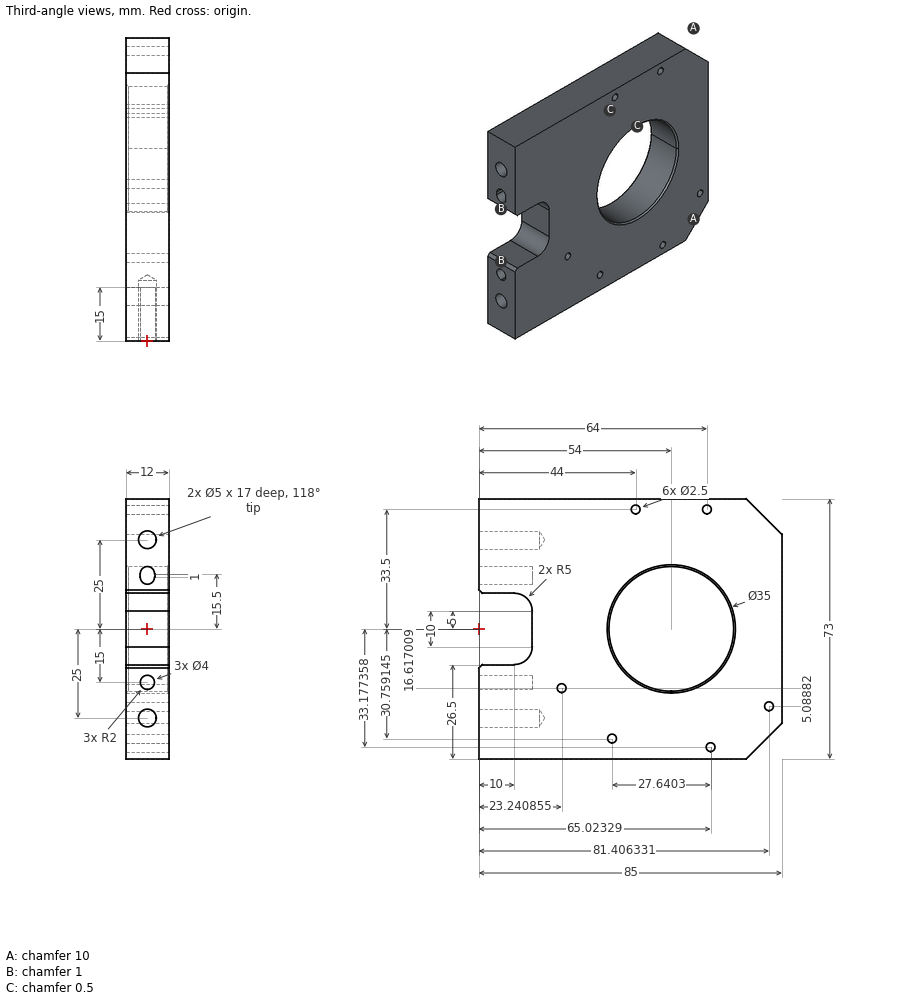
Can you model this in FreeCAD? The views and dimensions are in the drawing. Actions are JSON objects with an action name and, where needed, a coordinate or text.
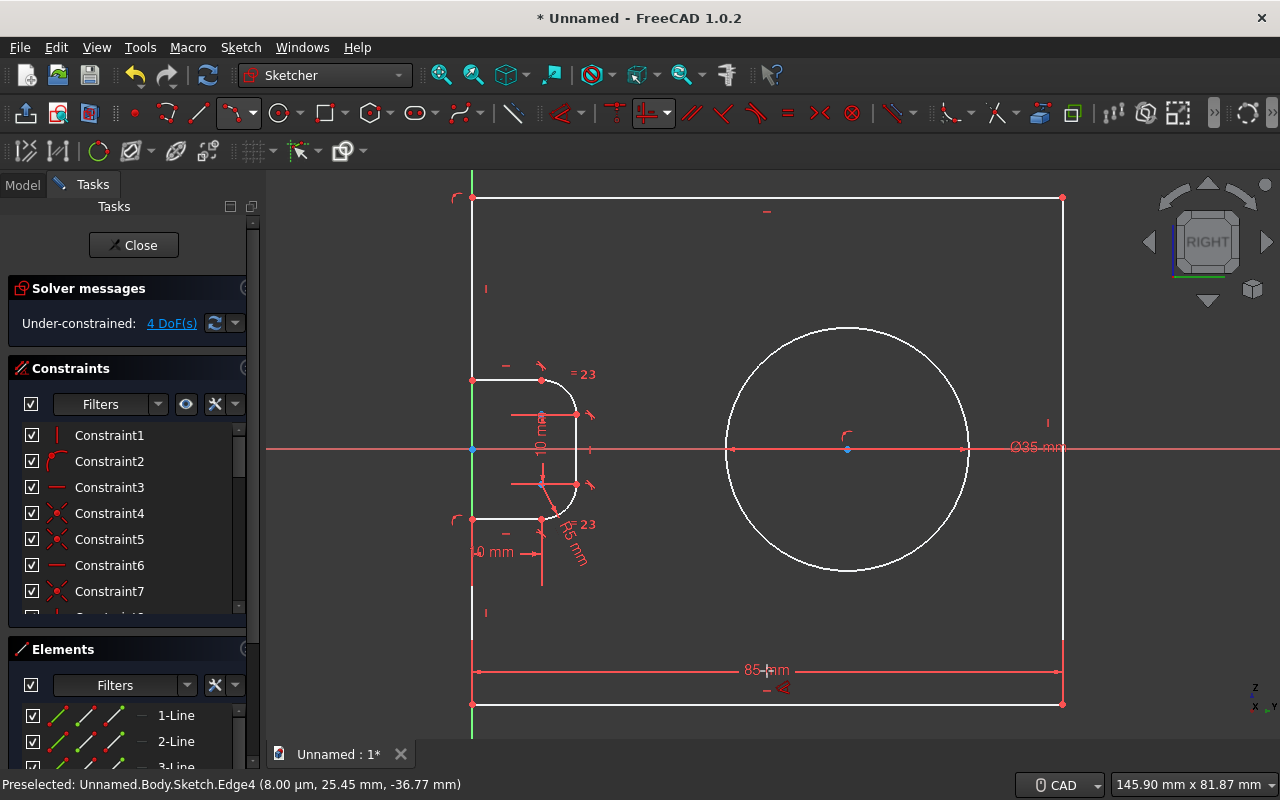
{"action": "left_click", "coordinate": [1063, 553]}
{"action": "left_click", "coordinate": [1097, 335]}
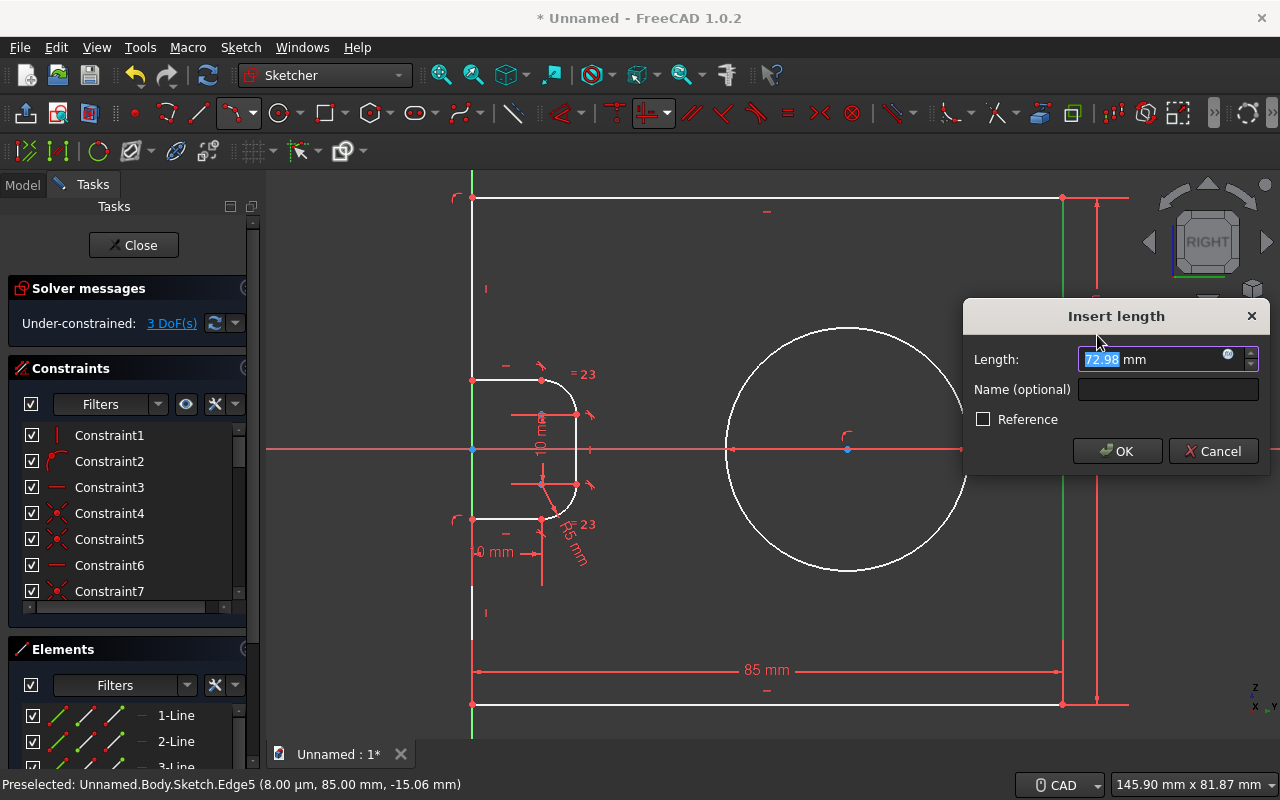
{"action": "type", "text": "73"}
{"action": "key", "text": "Return"}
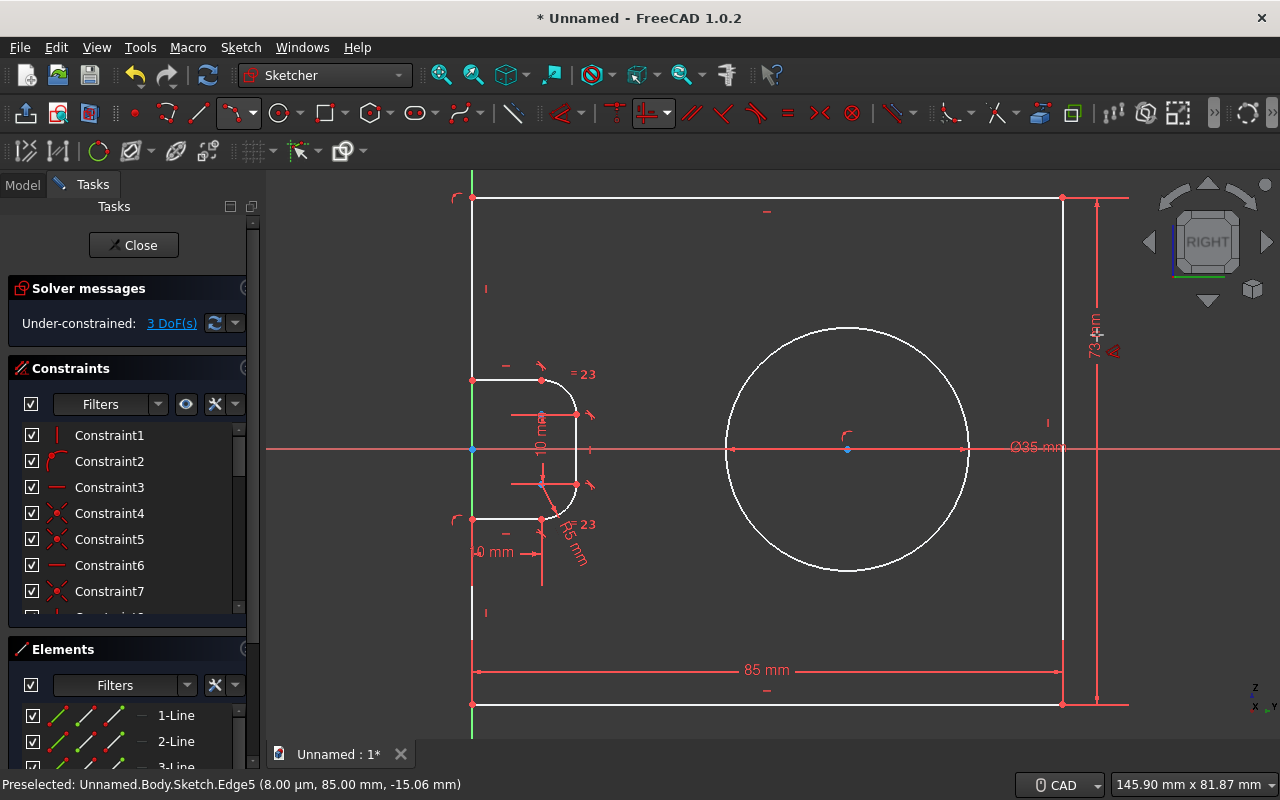
{"action": "left_click", "coordinate": [576, 415]}
{"action": "left_click", "coordinate": [438, 432]}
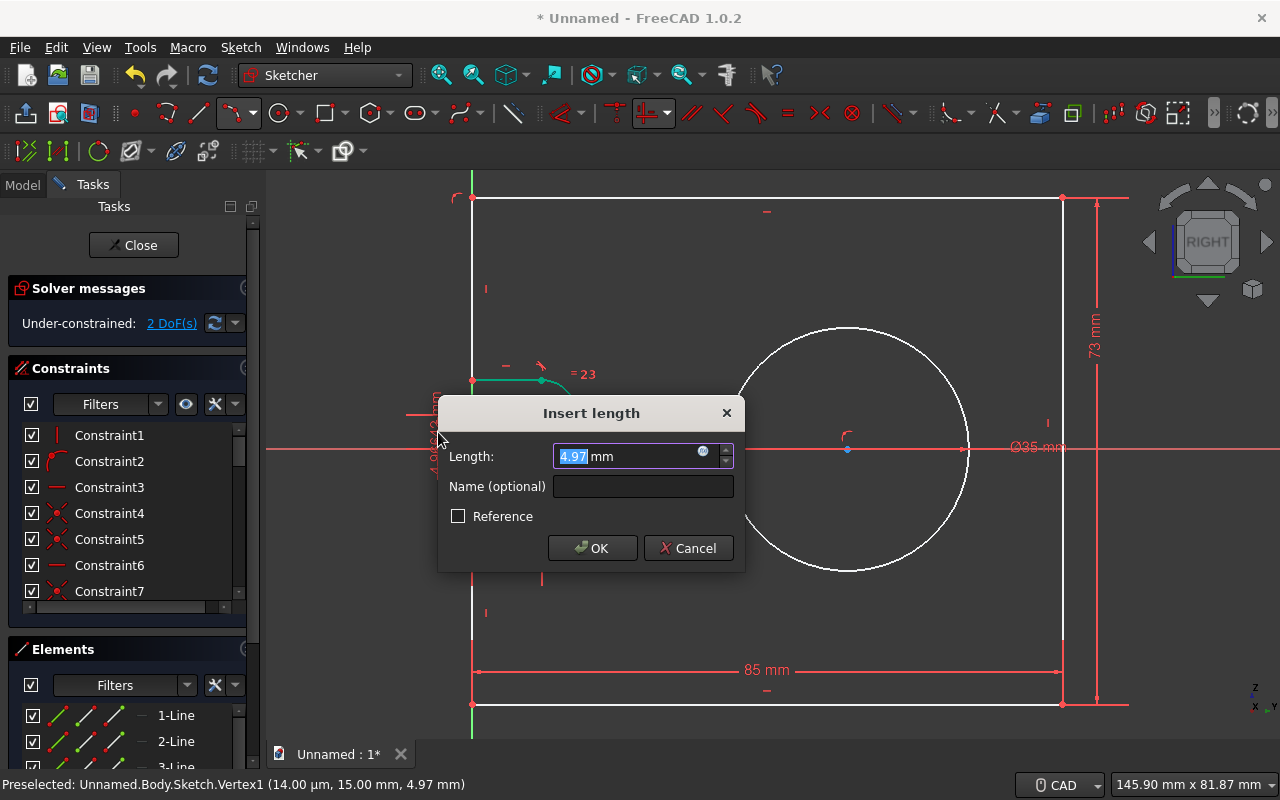
{"action": "type", "text": "5"}
{"action": "key", "text": "Return"}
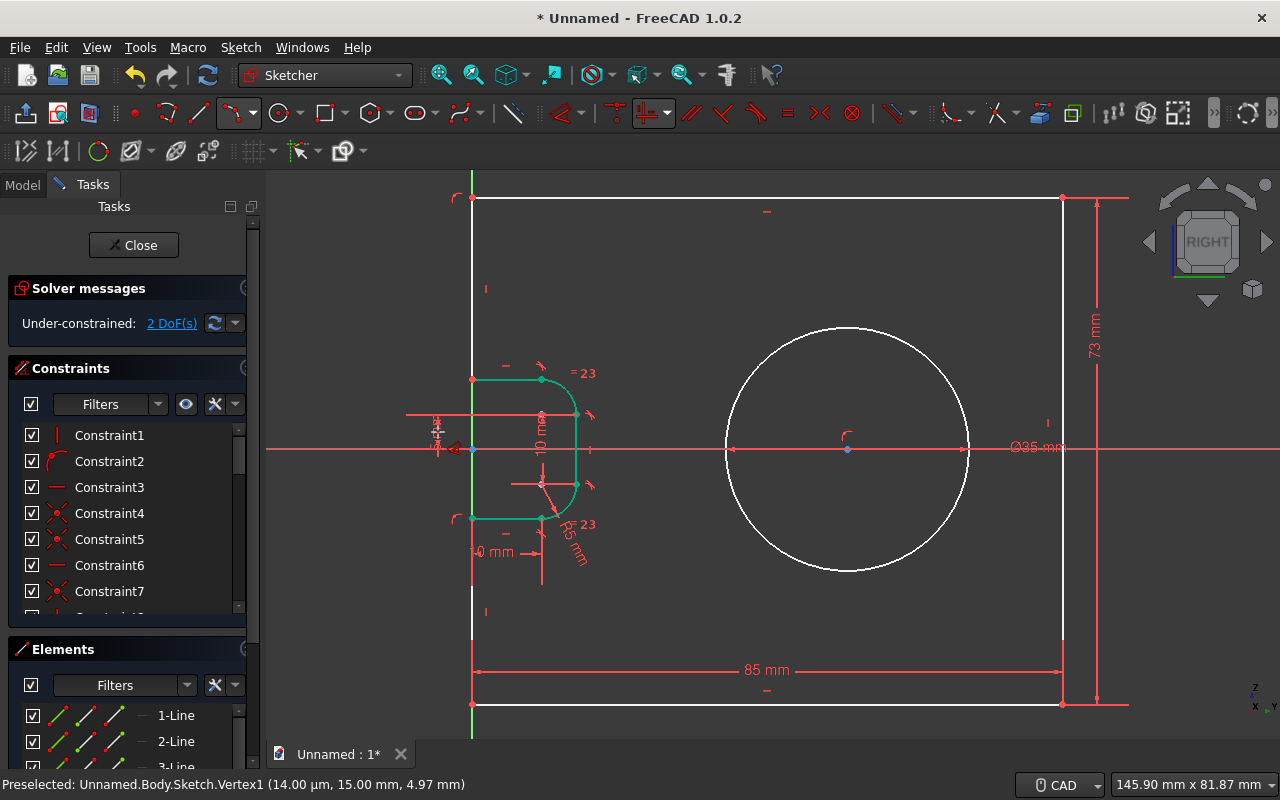
{"action": "left_click", "coordinate": [847, 449]}
{"action": "left_click", "coordinate": [660, 483]}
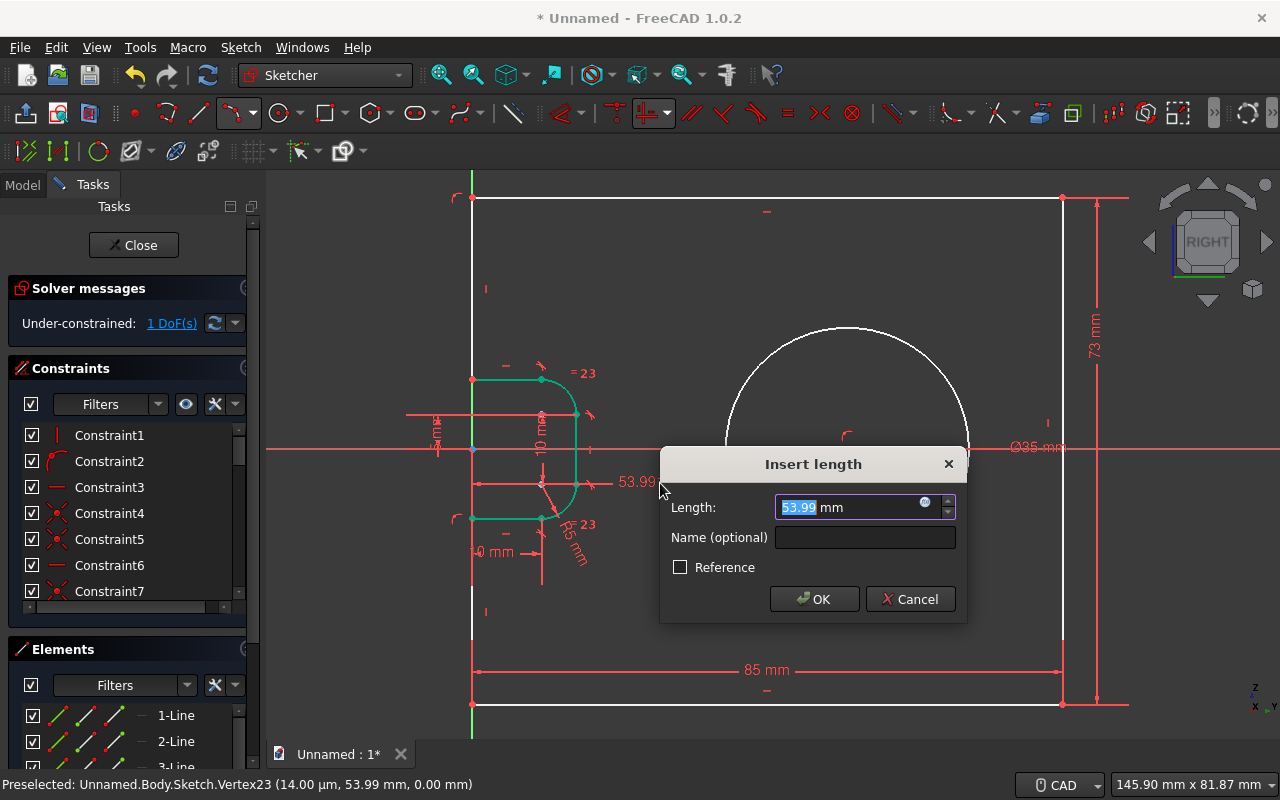
{"action": "type", "text": "54"}
{"action": "key", "text": "Return"}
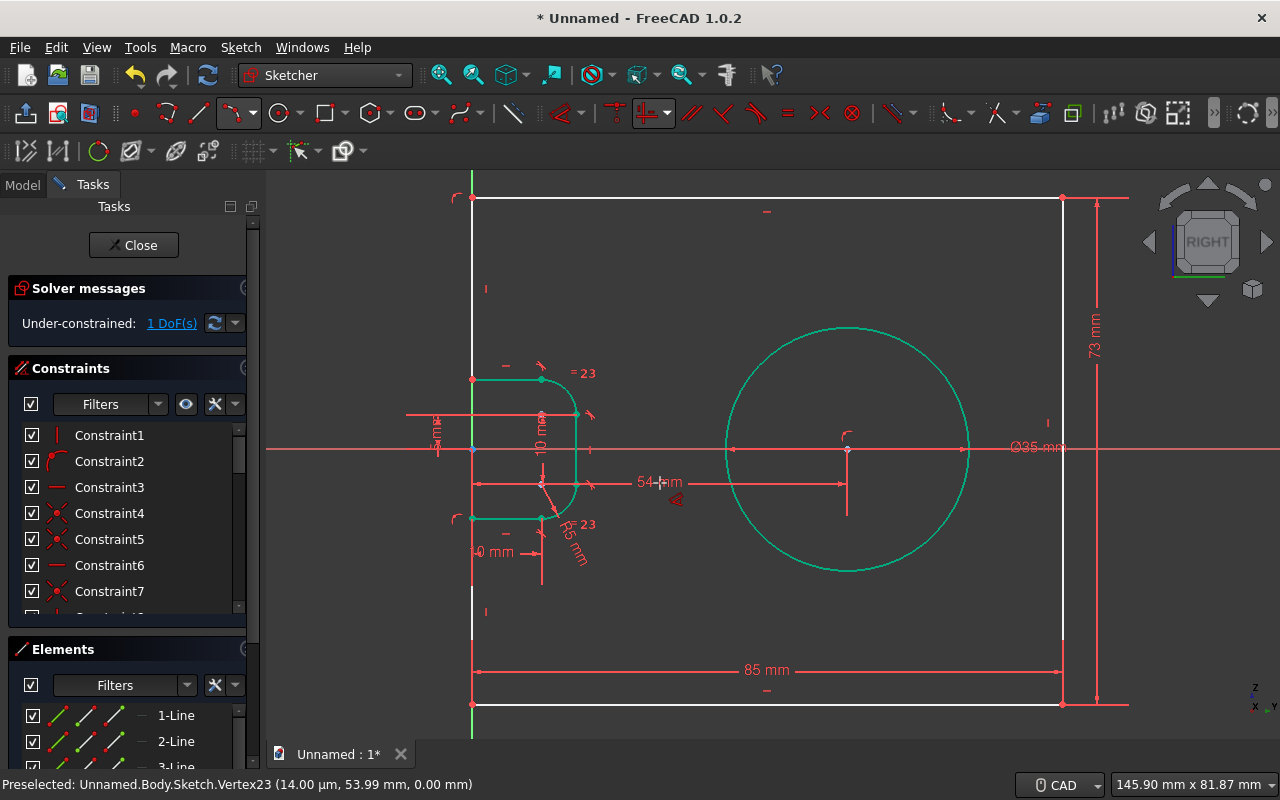
{"action": "left_click", "coordinate": [472, 575]}
{"action": "left_click", "coordinate": [438, 612]}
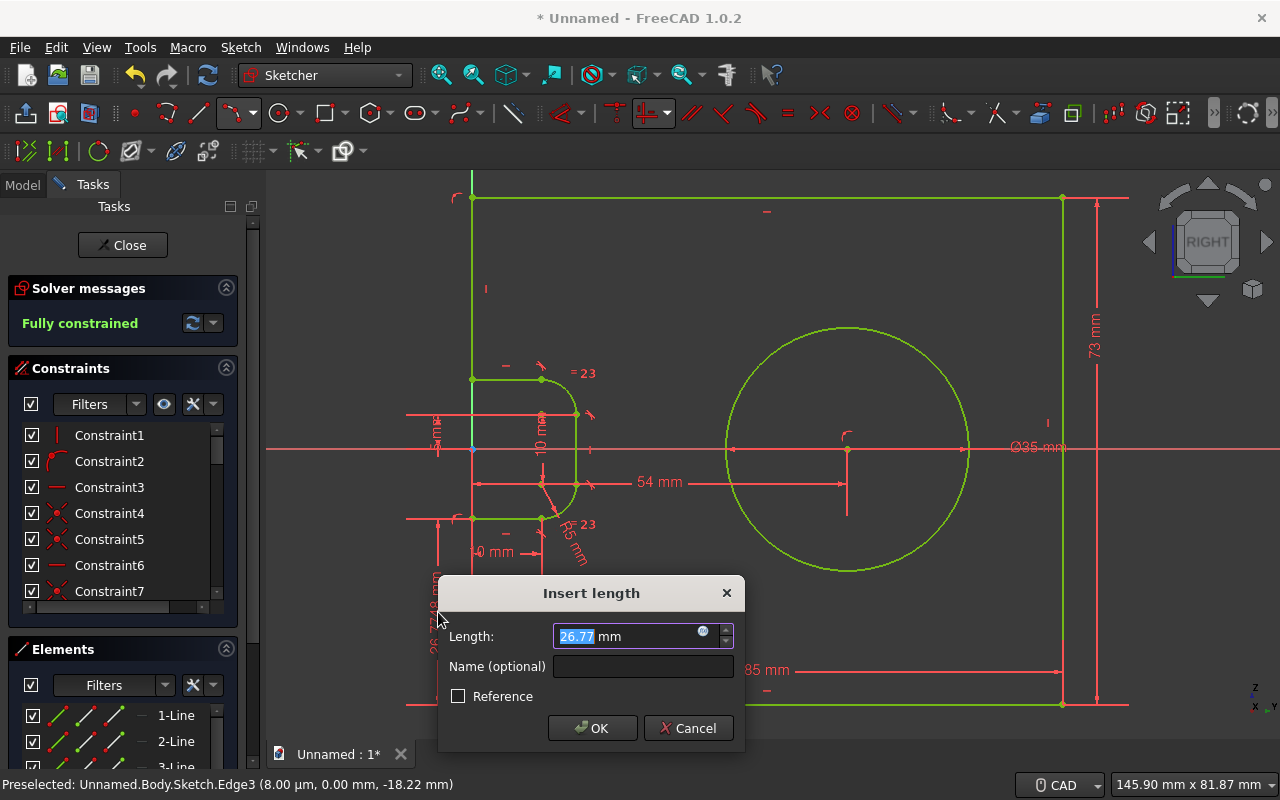
{"action": "type", "text": "26.5"}
{"action": "key", "text": "Return"}
{"action": "key", "text": "Escape"}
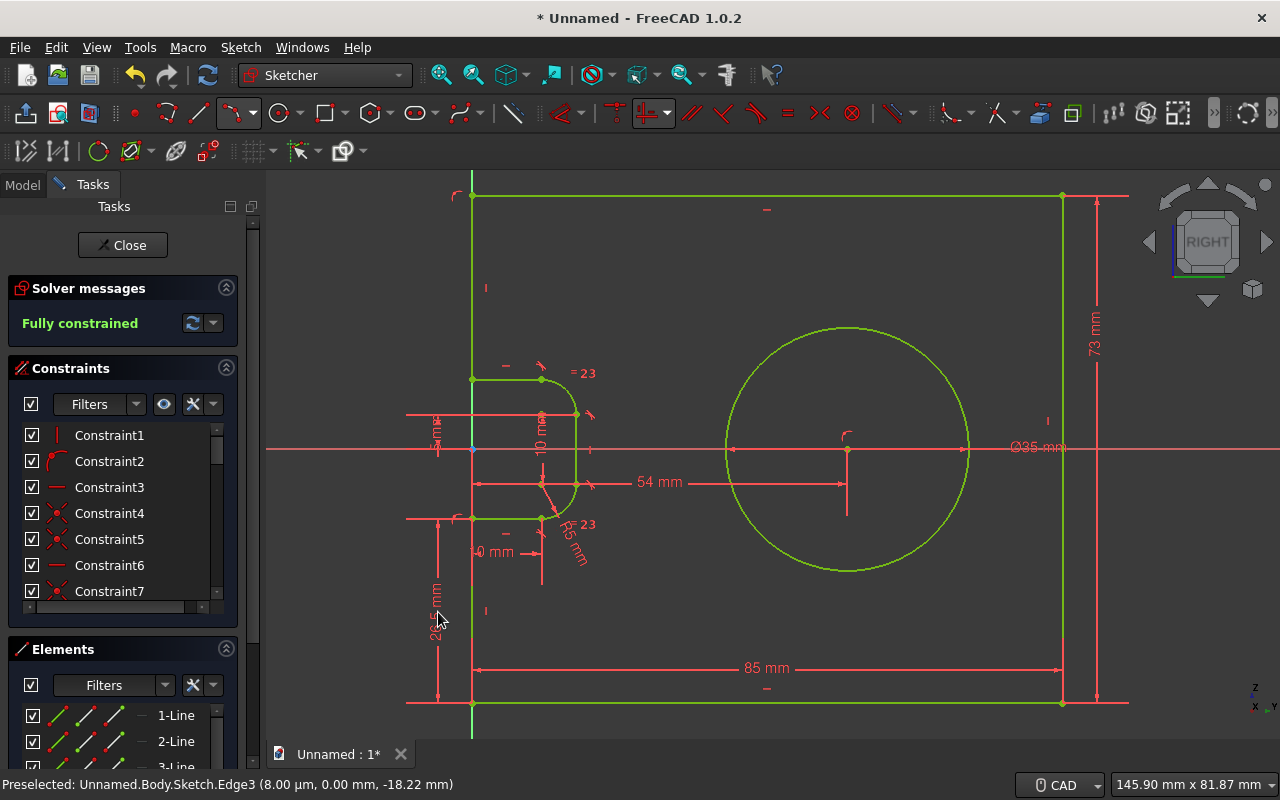
{"action": "left_click", "coordinate": [123, 245]}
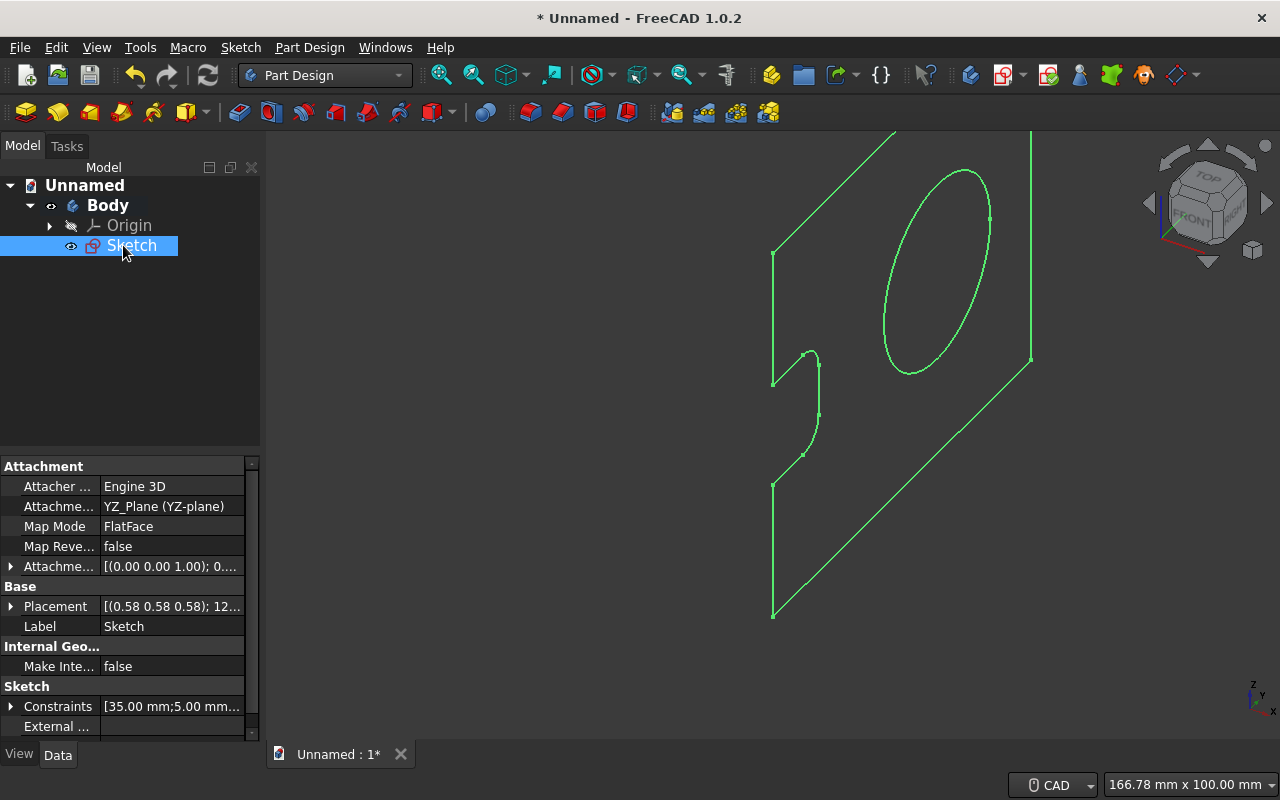
{"action": "left_click", "coordinate": [26, 112]}